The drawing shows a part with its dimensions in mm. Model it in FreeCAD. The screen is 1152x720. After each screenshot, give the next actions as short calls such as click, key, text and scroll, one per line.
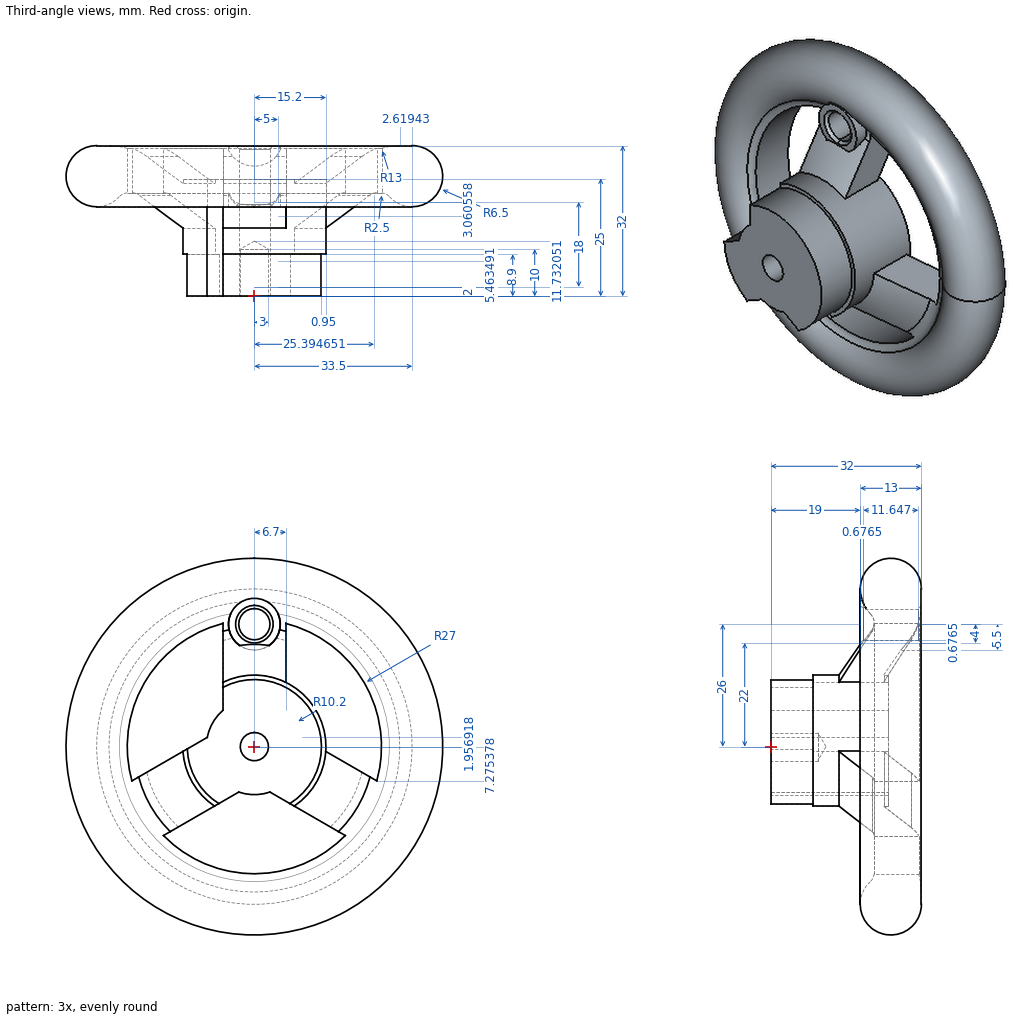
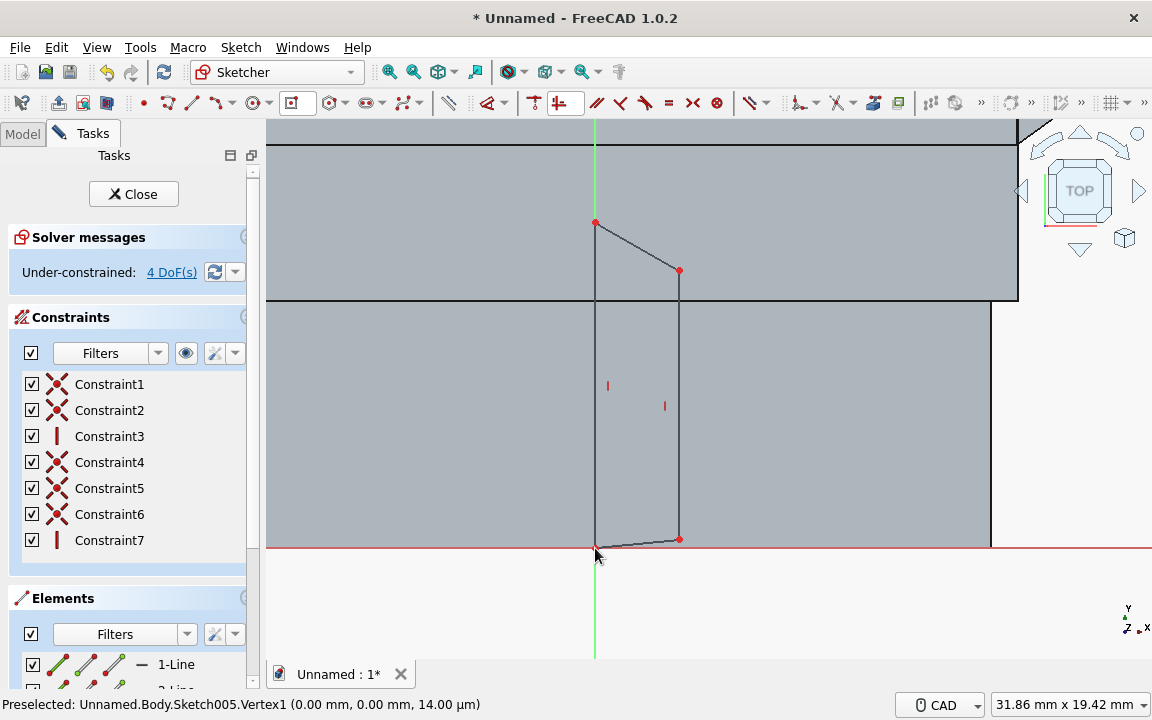
click(620, 546)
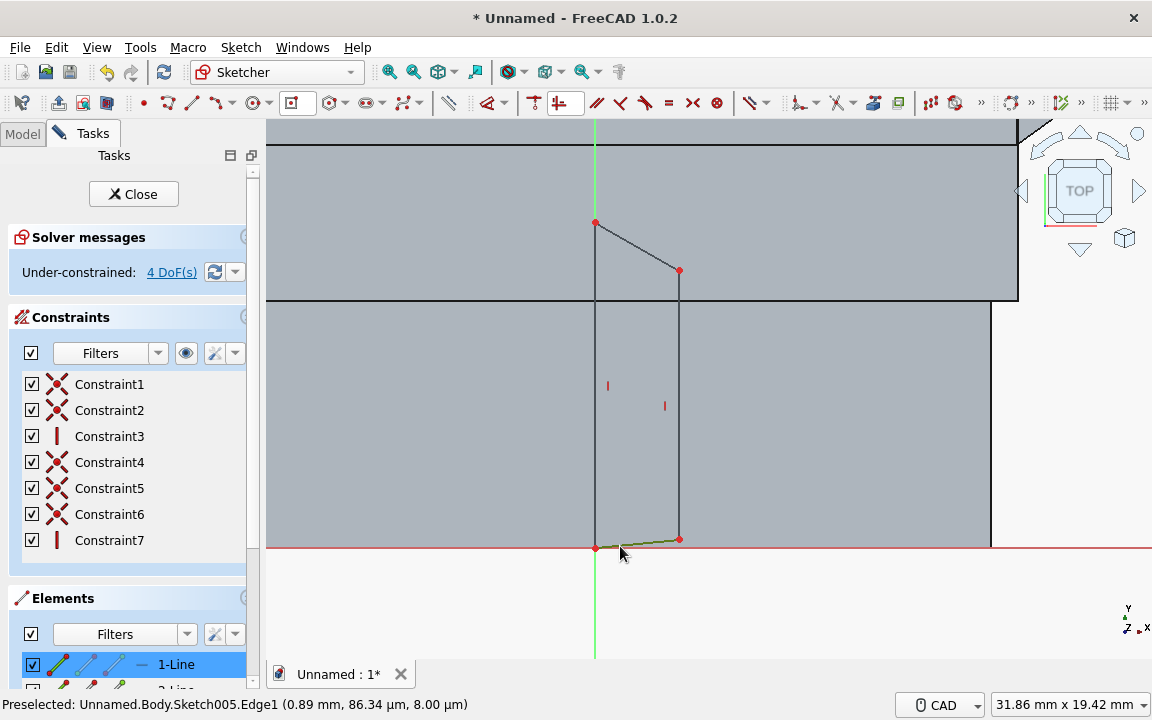
key(h)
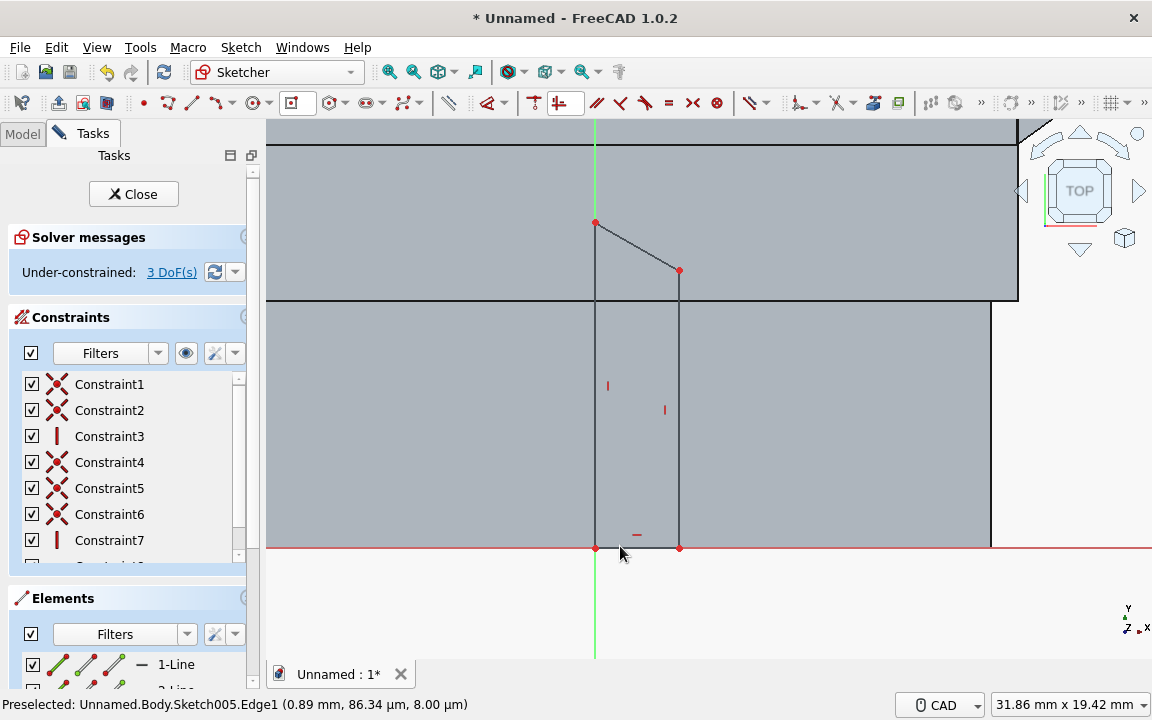
click(488, 104)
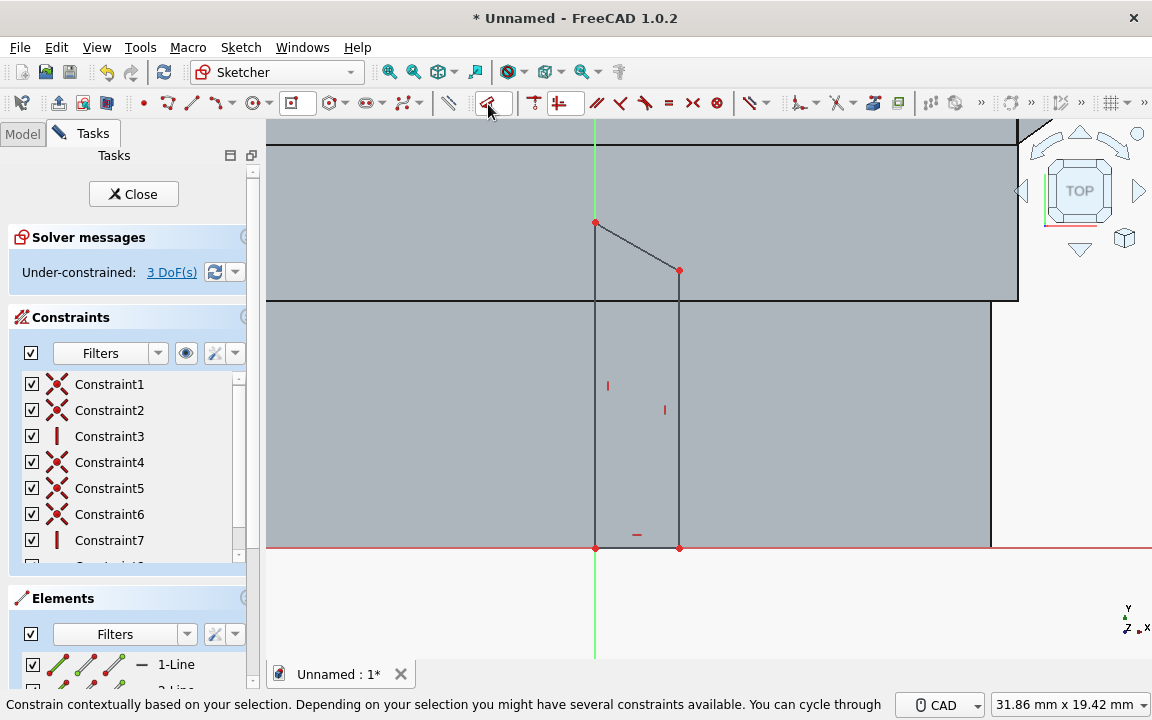
click(620, 548)
click(637, 582)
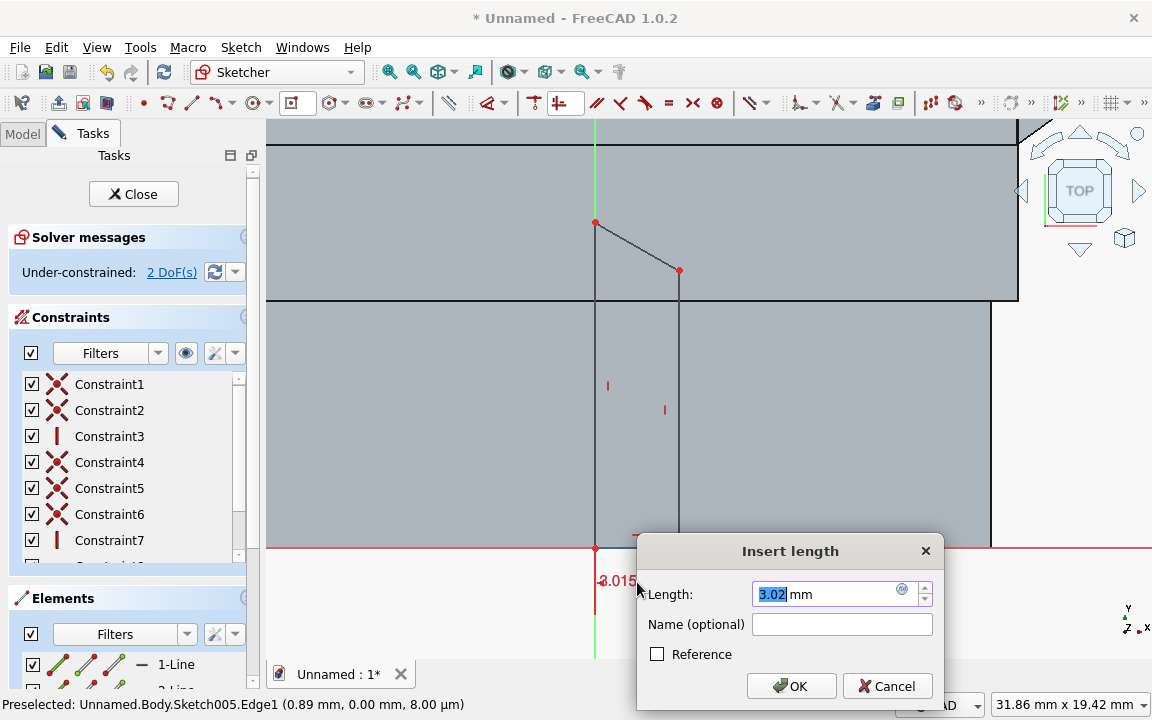
text(3)
key(Return)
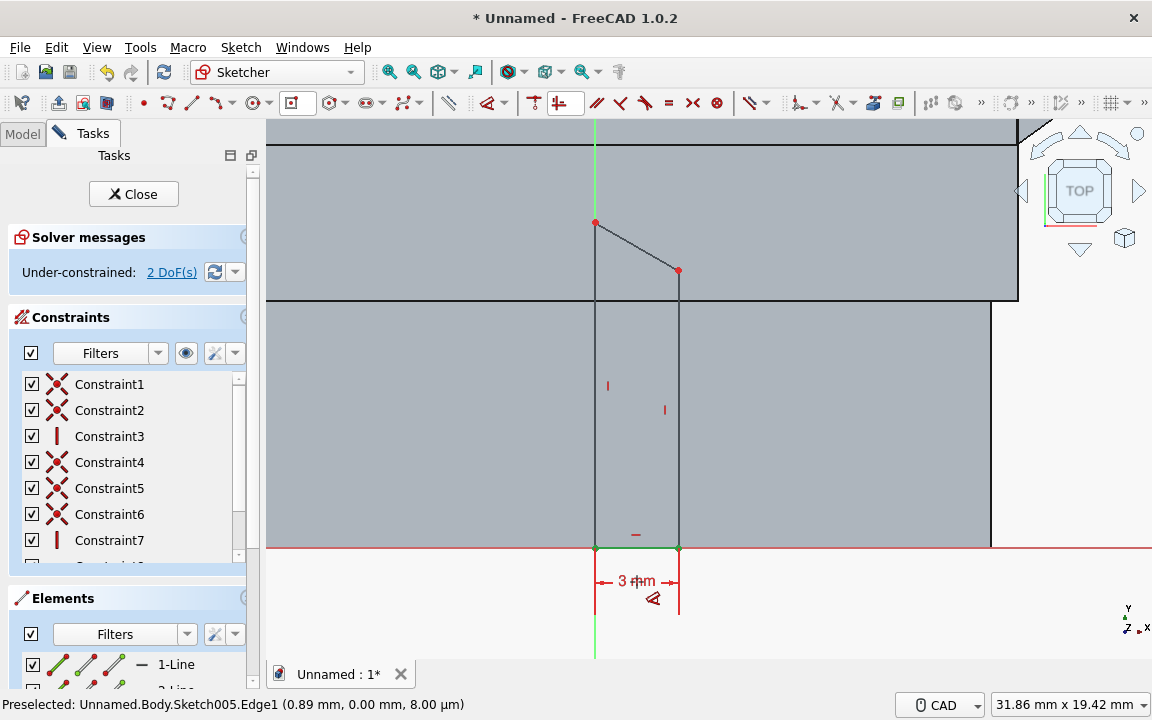
click(679, 465)
click(713, 410)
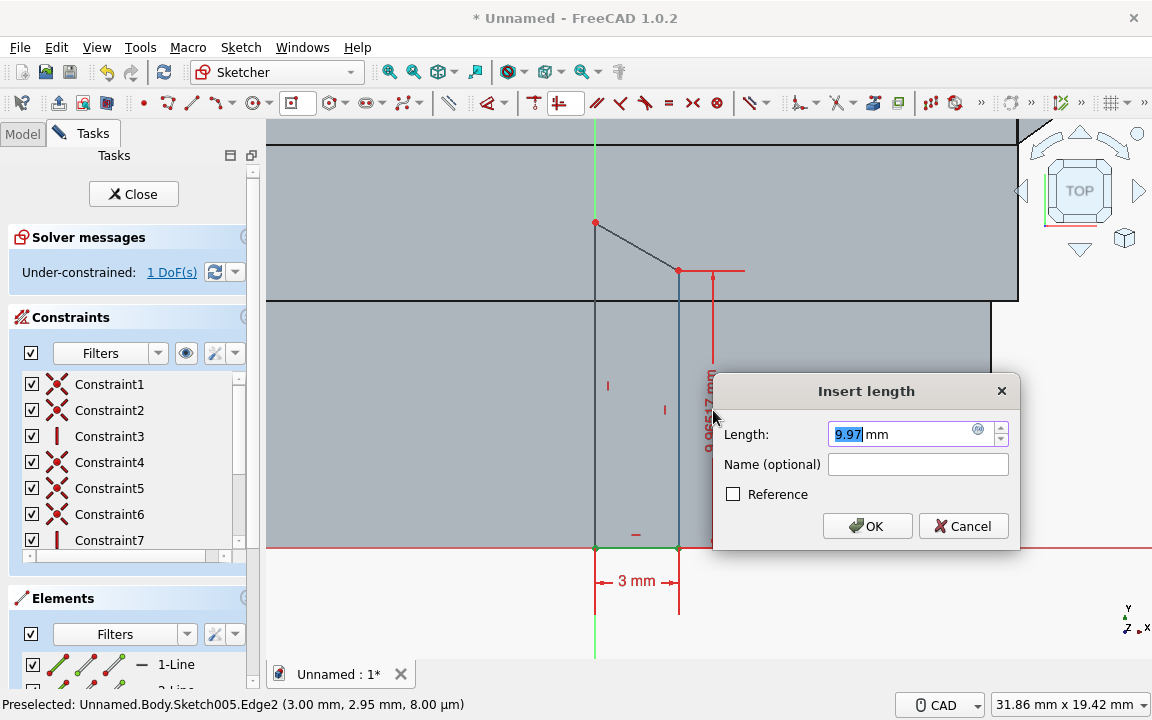
text(10)
key(Return)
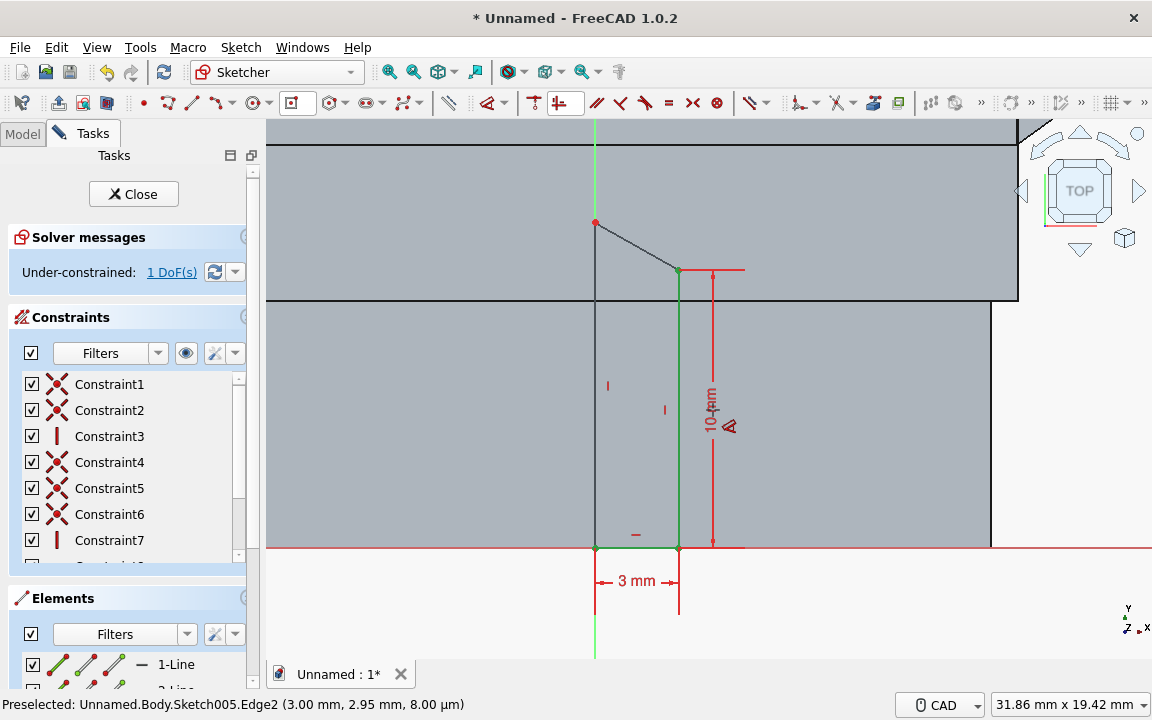
click(595, 321)
click(561, 386)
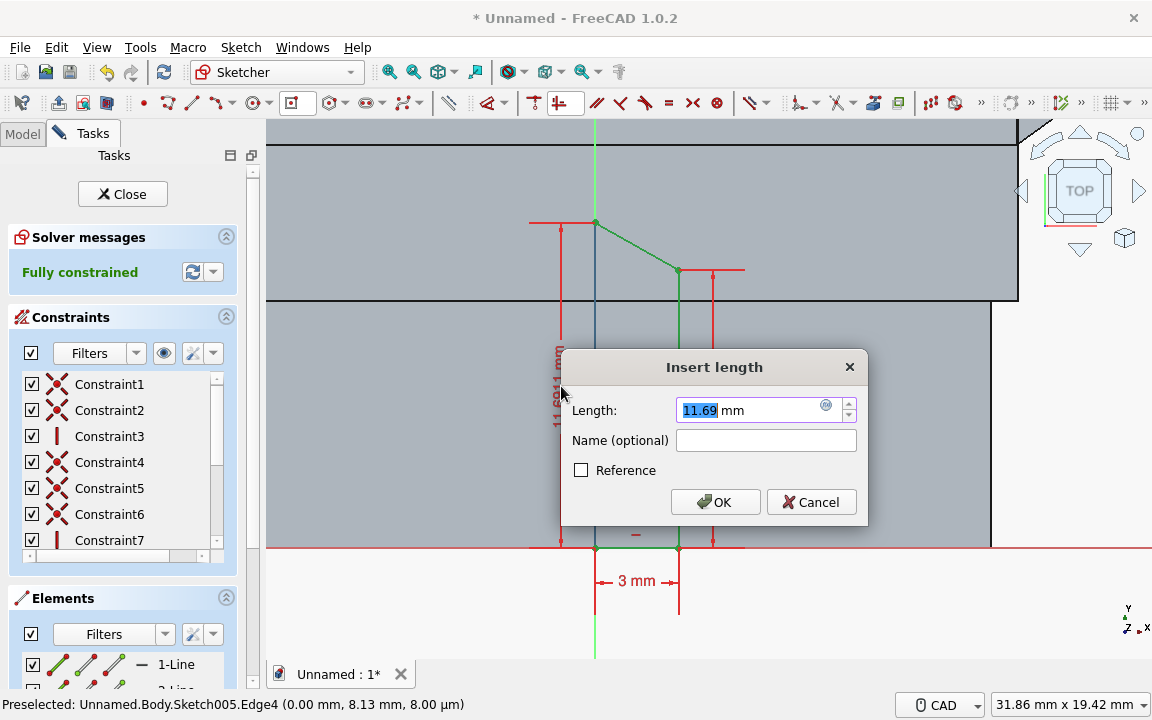
text(11.732051)
key(Return)
key(Escape)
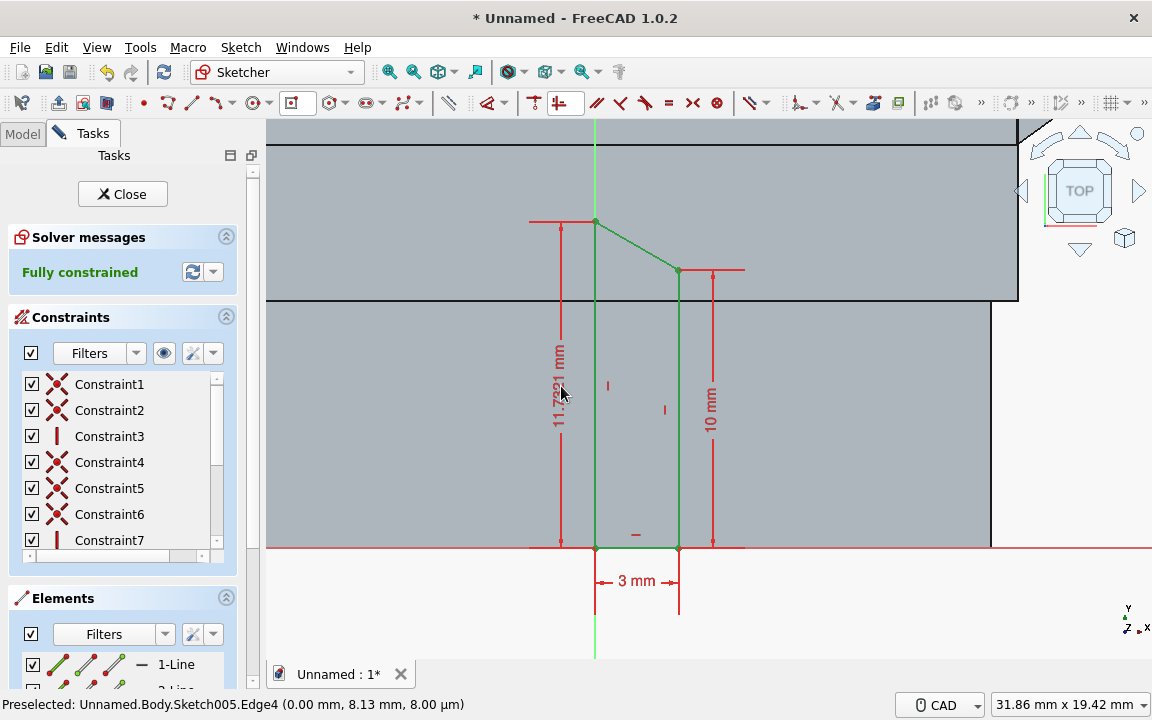
click(123, 194)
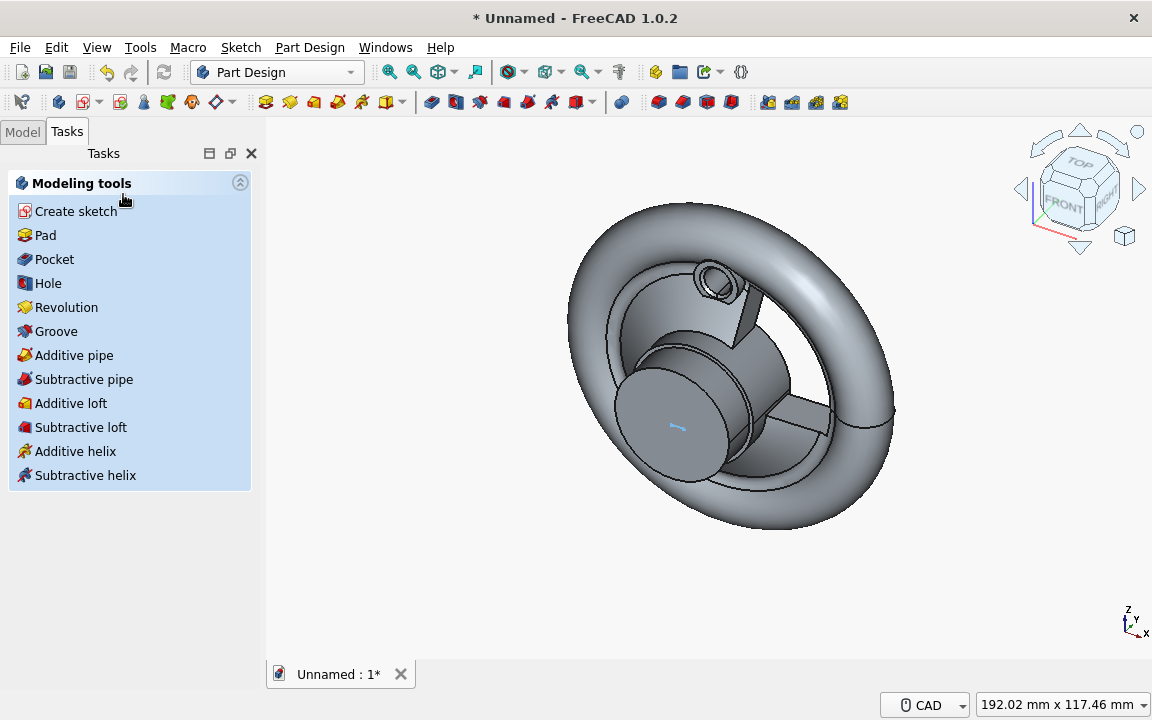
click(480, 102)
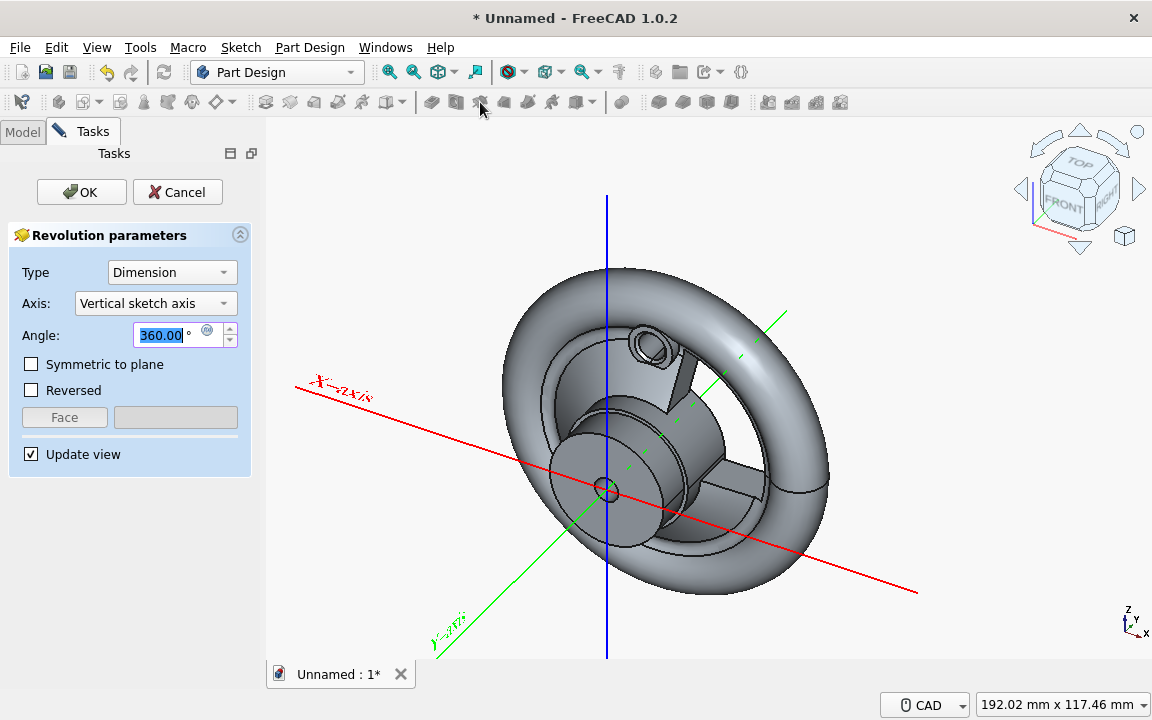
click(82, 192)